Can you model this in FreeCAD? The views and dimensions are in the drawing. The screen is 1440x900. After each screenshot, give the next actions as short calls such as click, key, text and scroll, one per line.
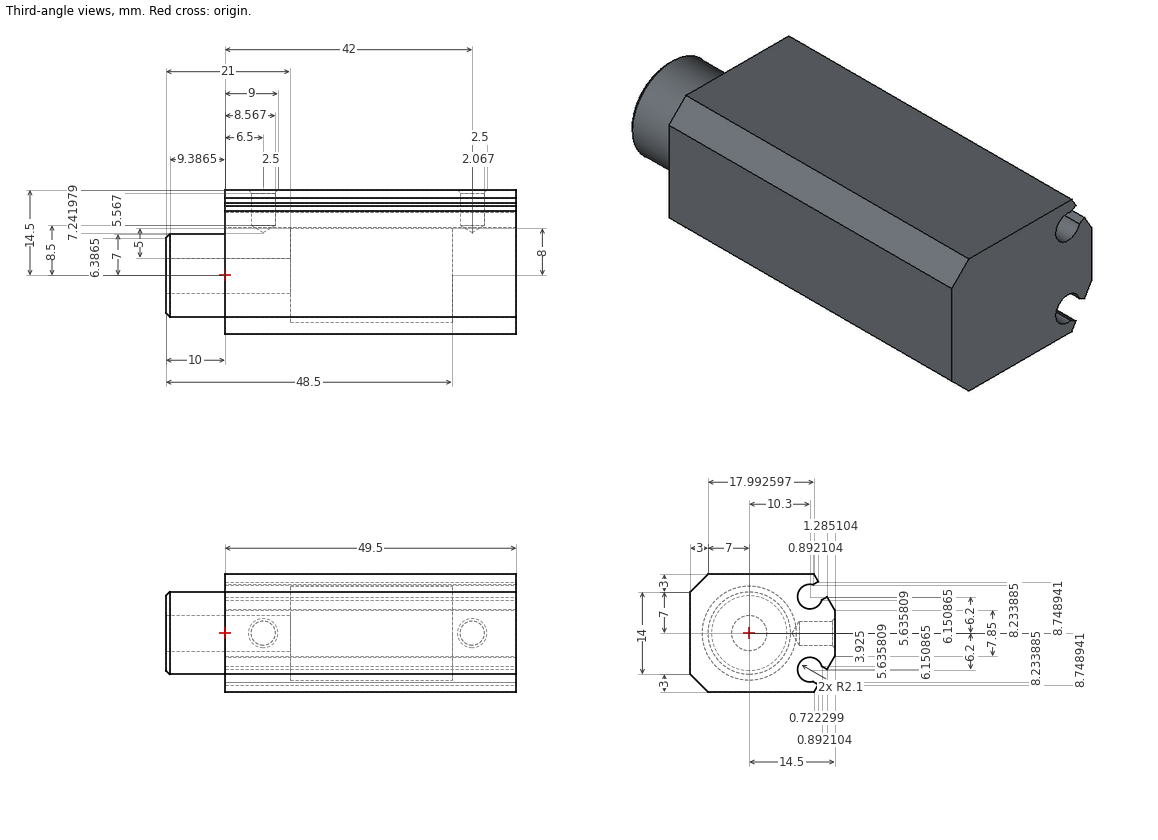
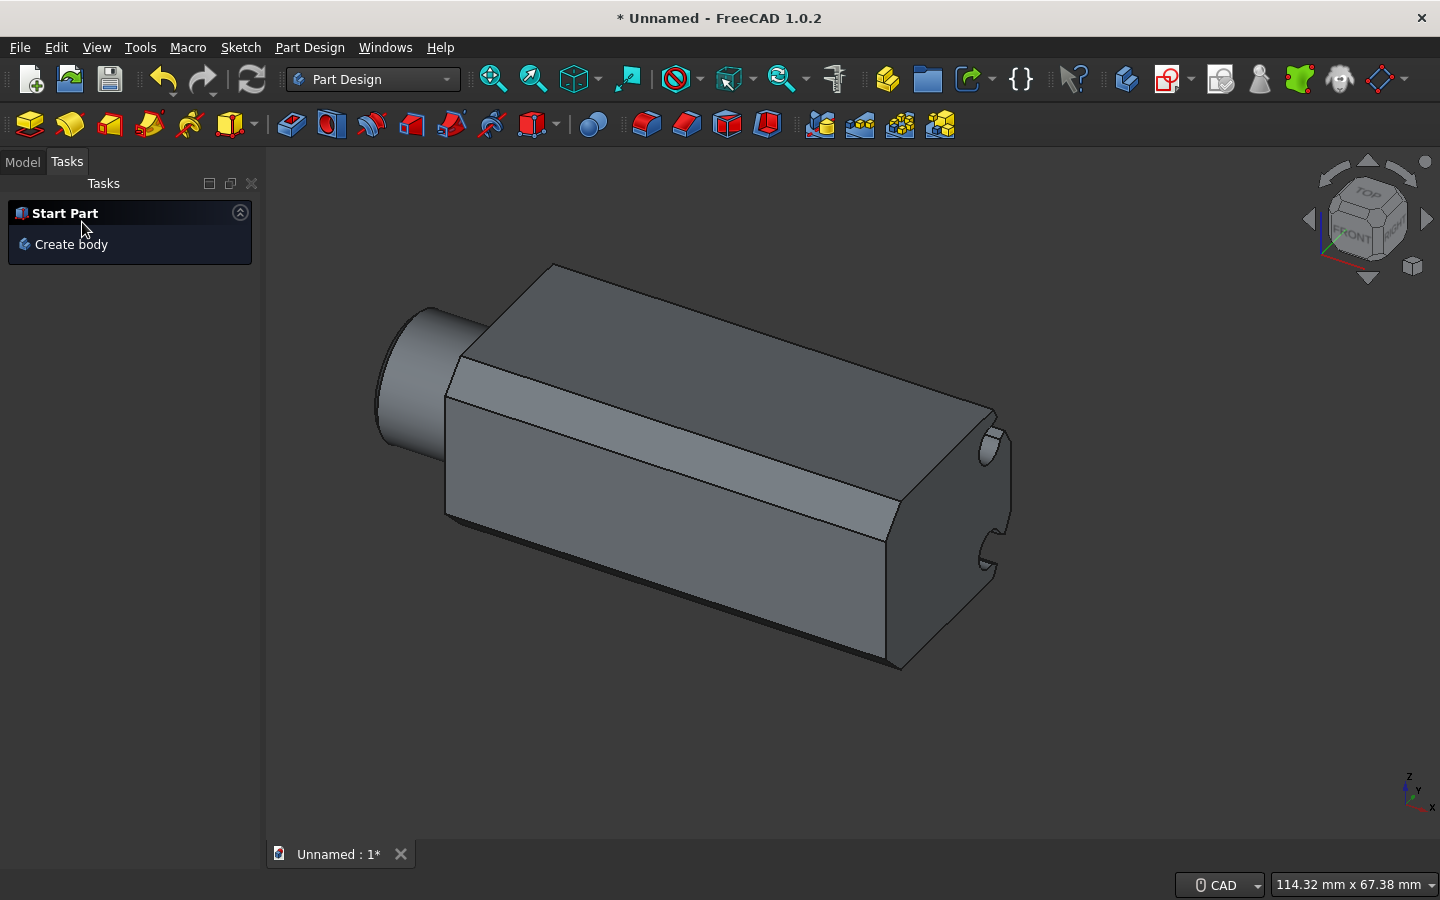
click(1168, 80)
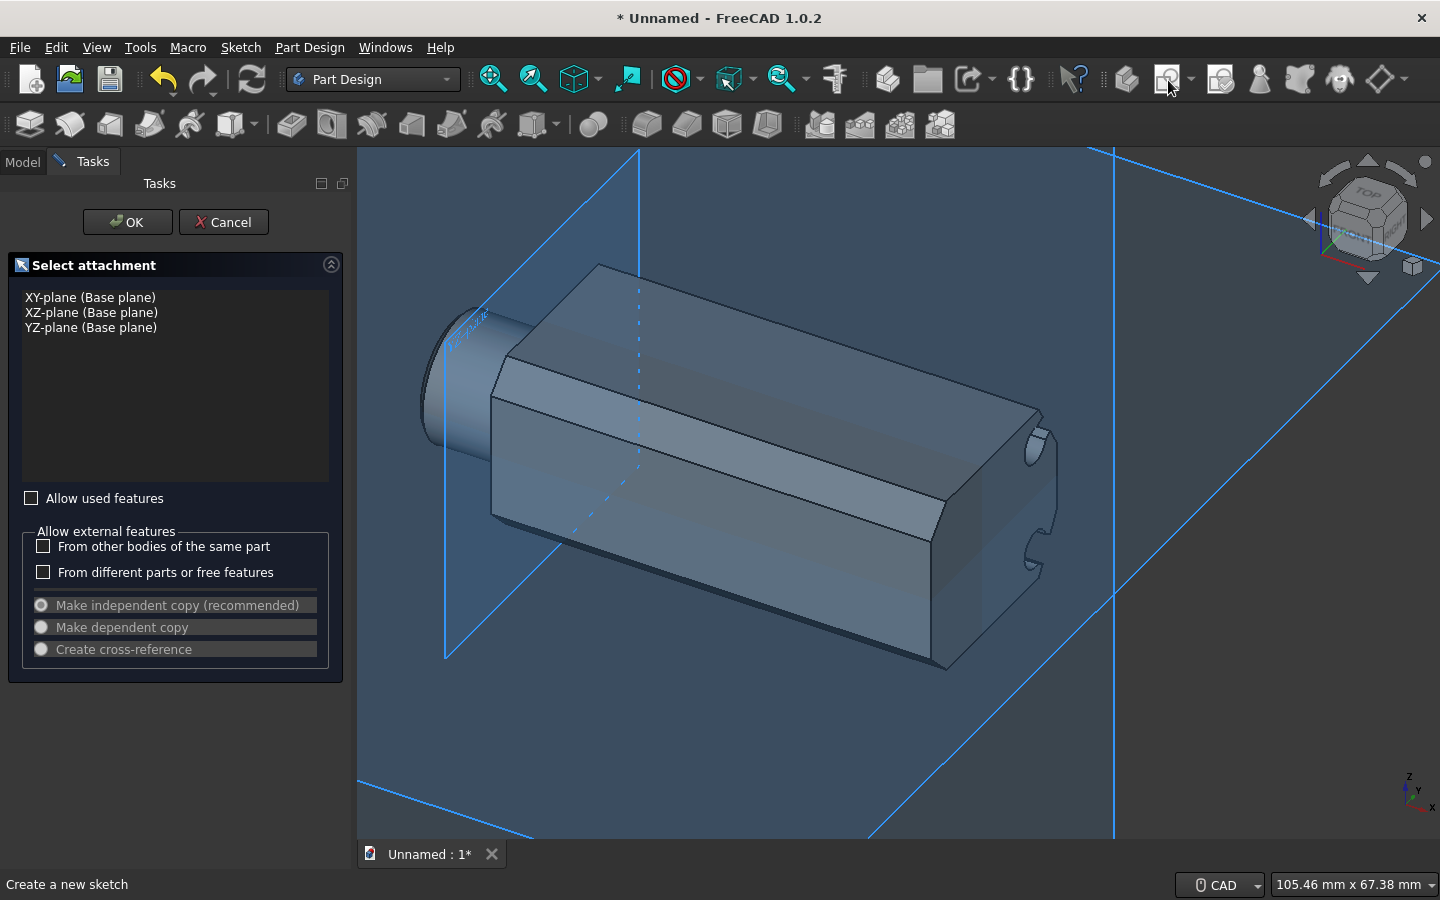
click(82, 298)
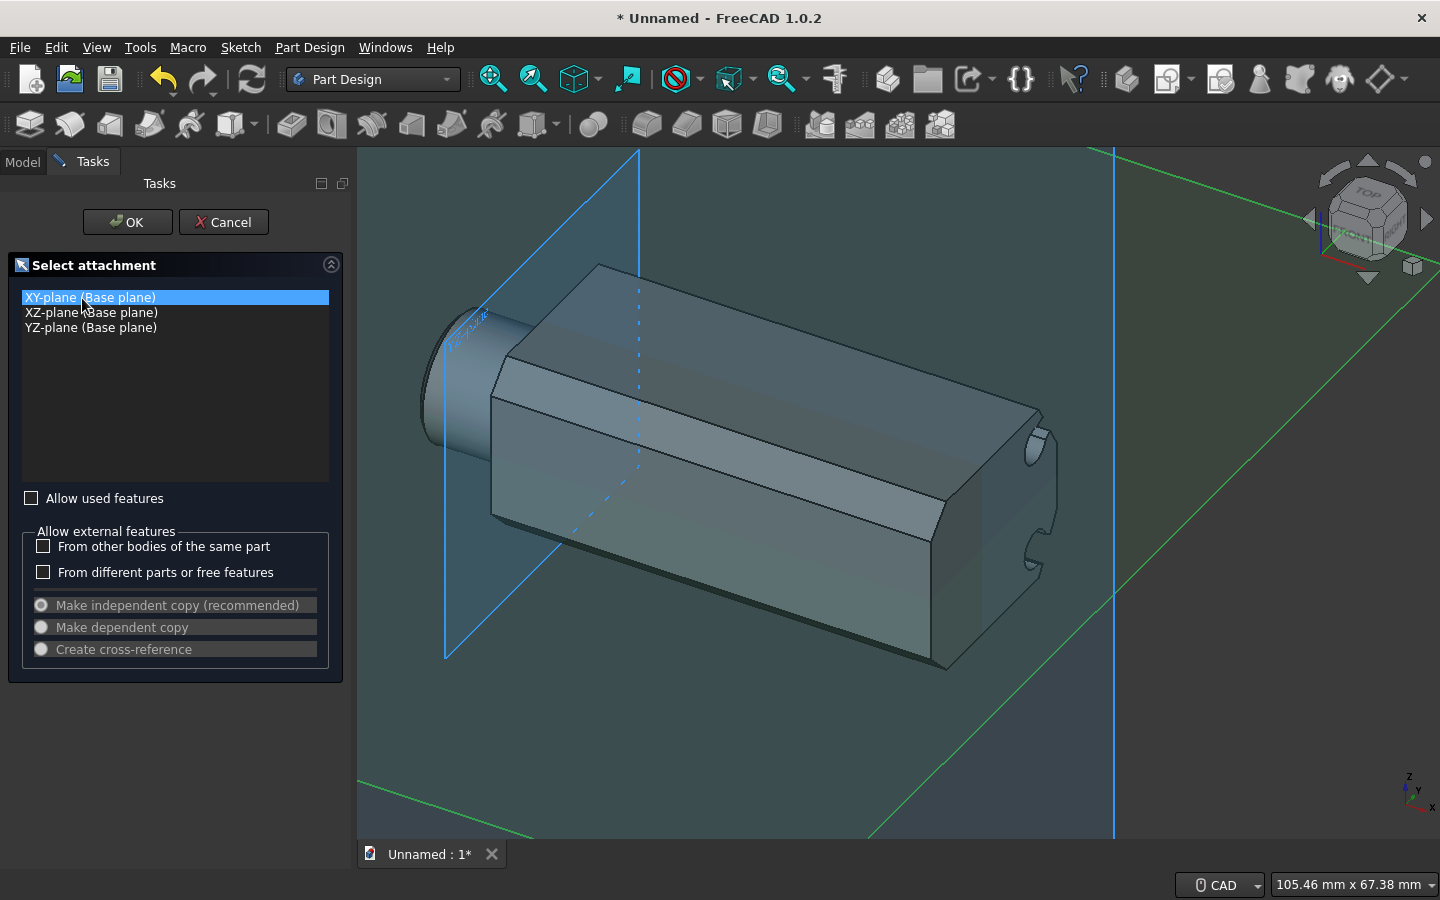
click(128, 222)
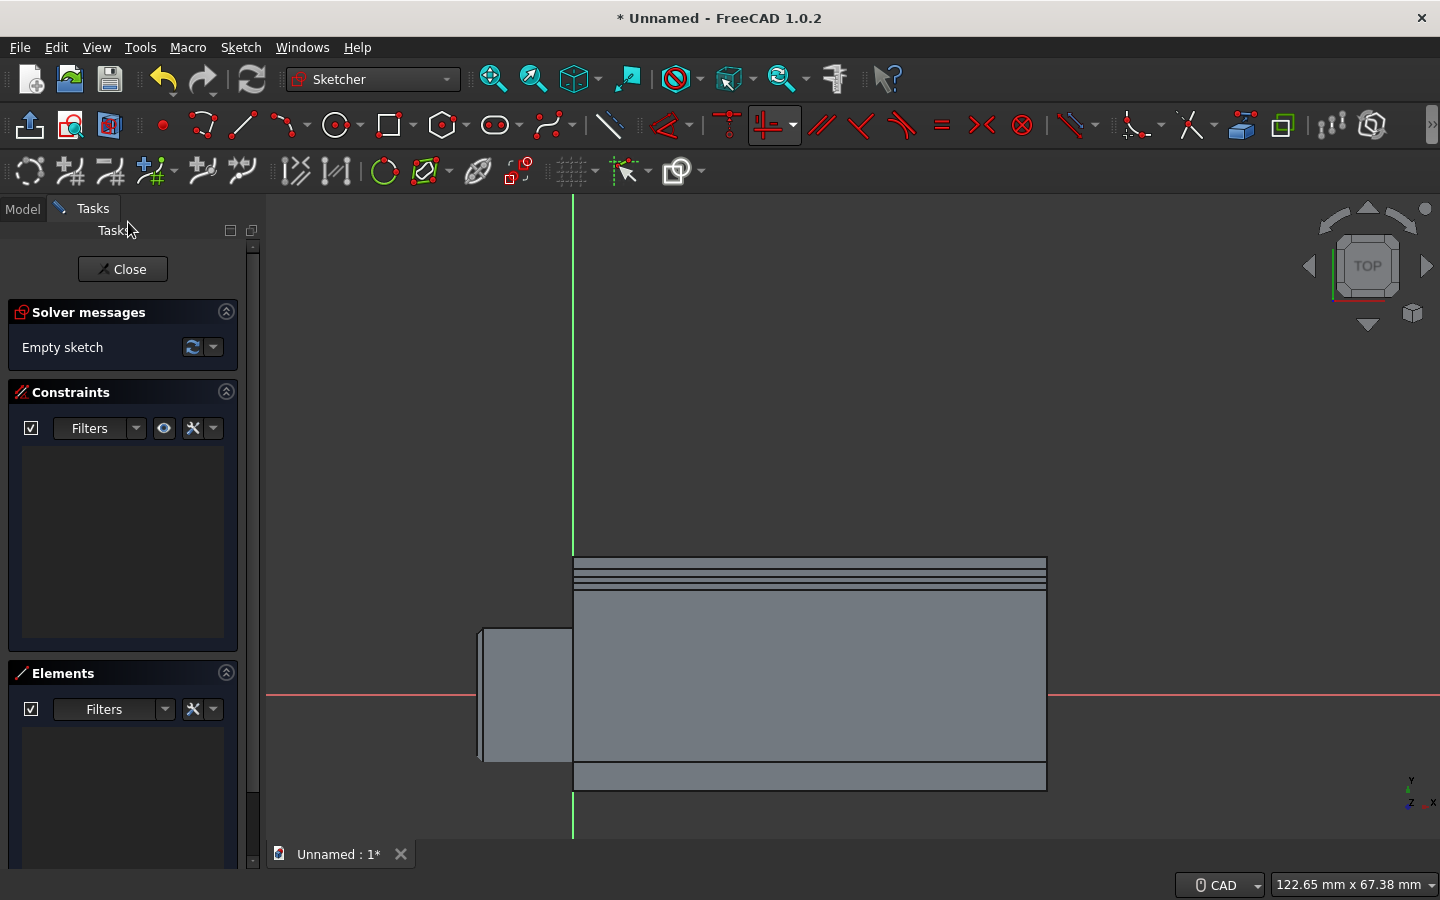
click(110, 126)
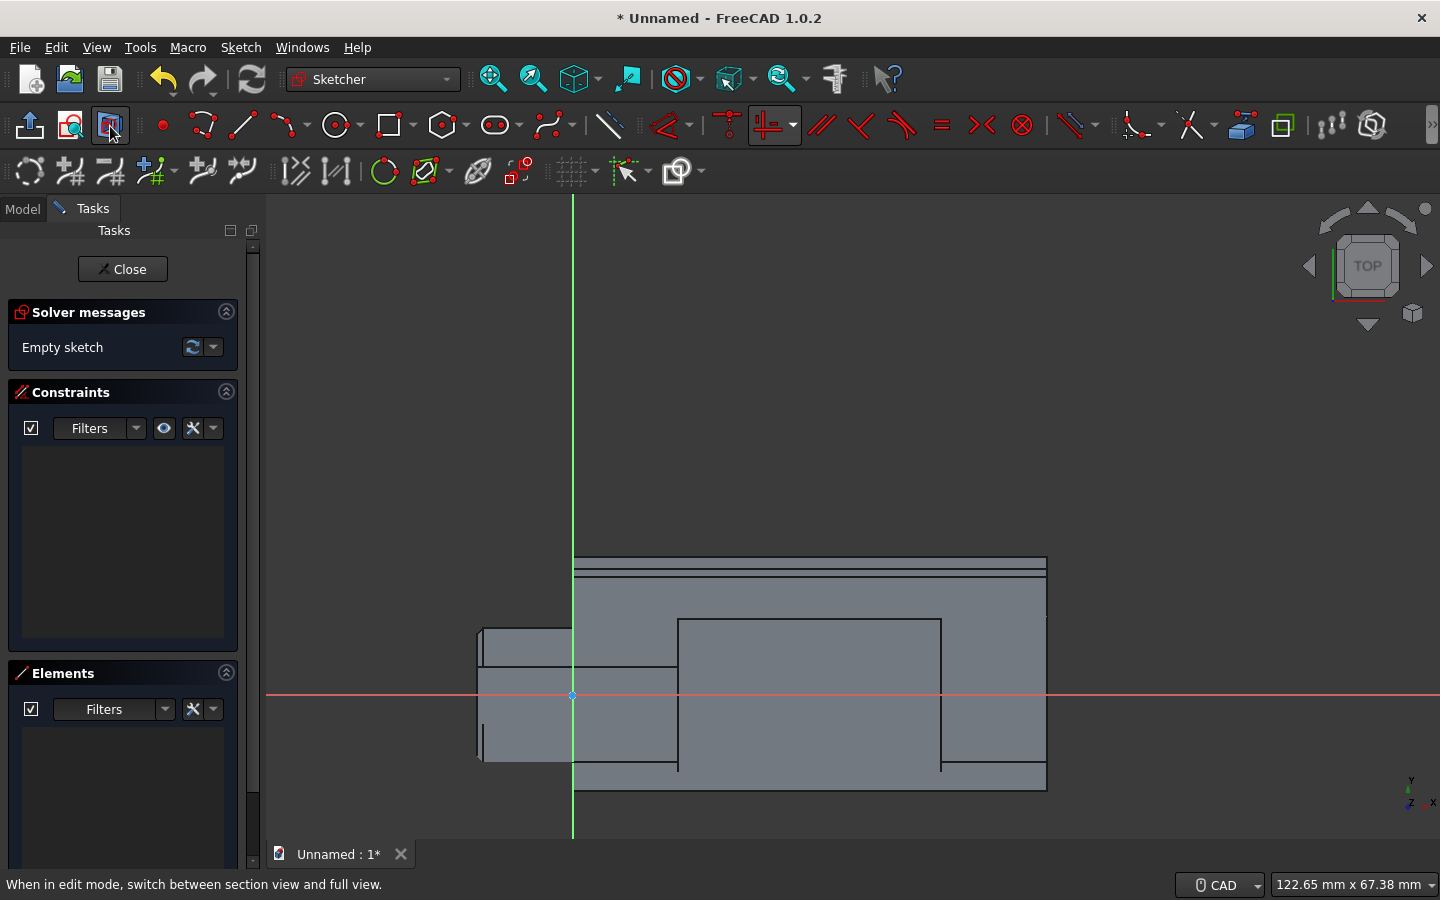
scroll(518, 668, up, 5)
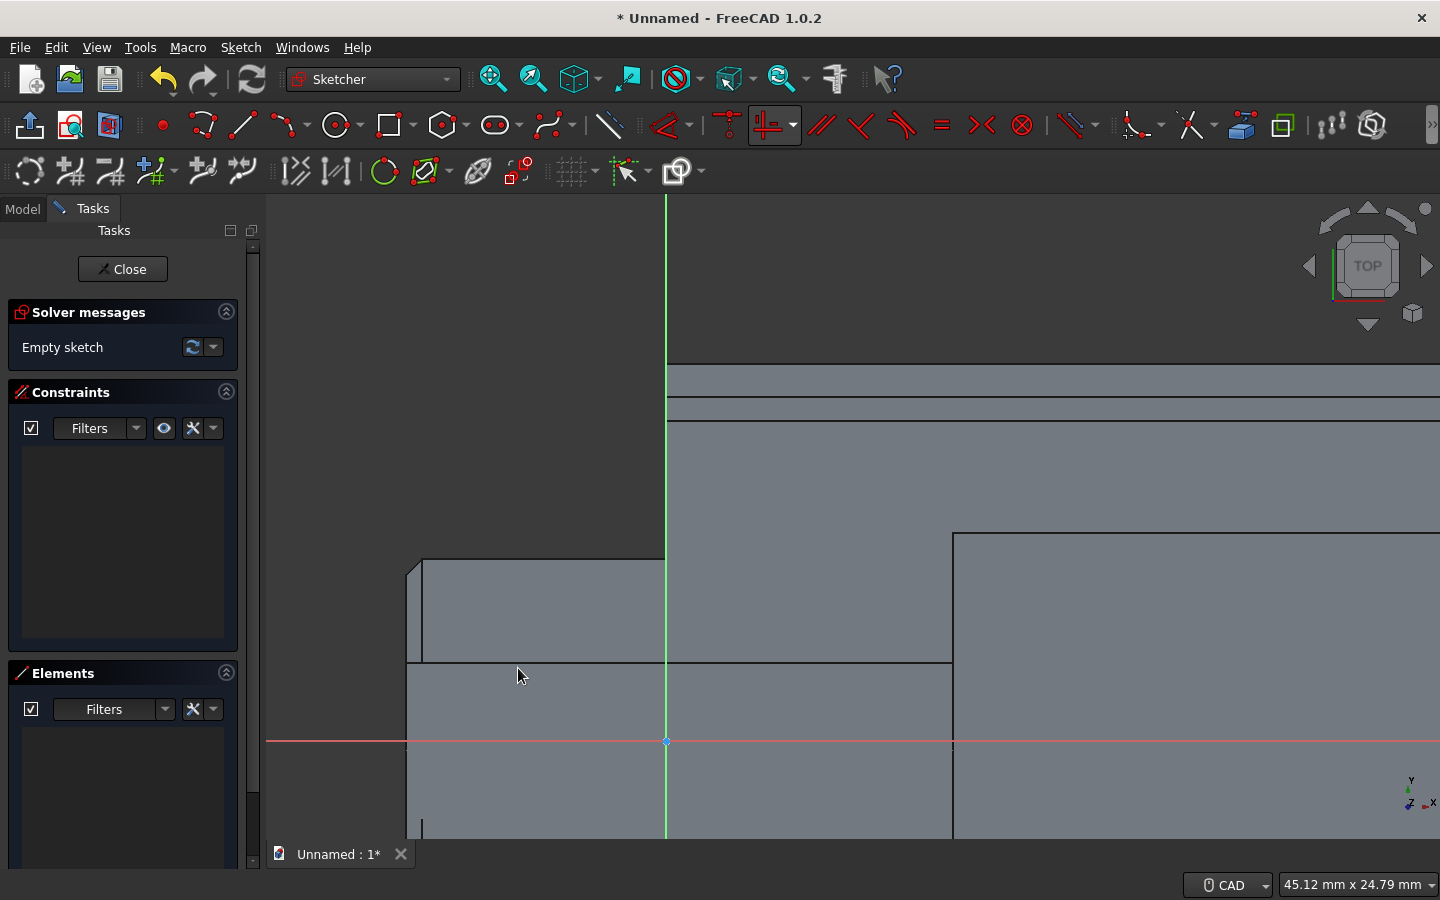
click(204, 126)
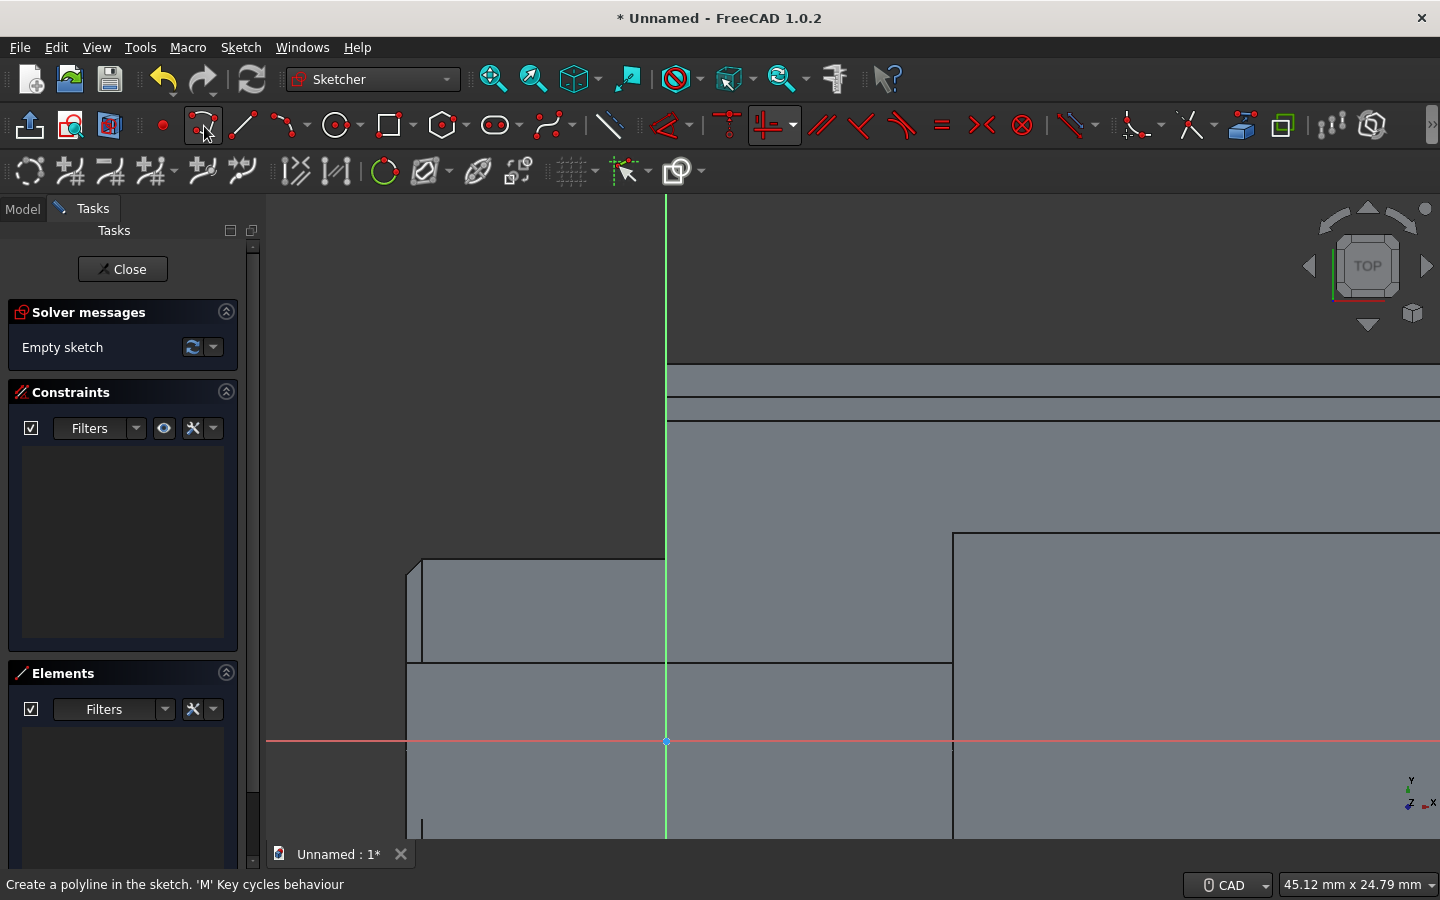
click(836, 552)
click(889, 520)
click(889, 375)
click(901, 364)
click(836, 364)
click(836, 553)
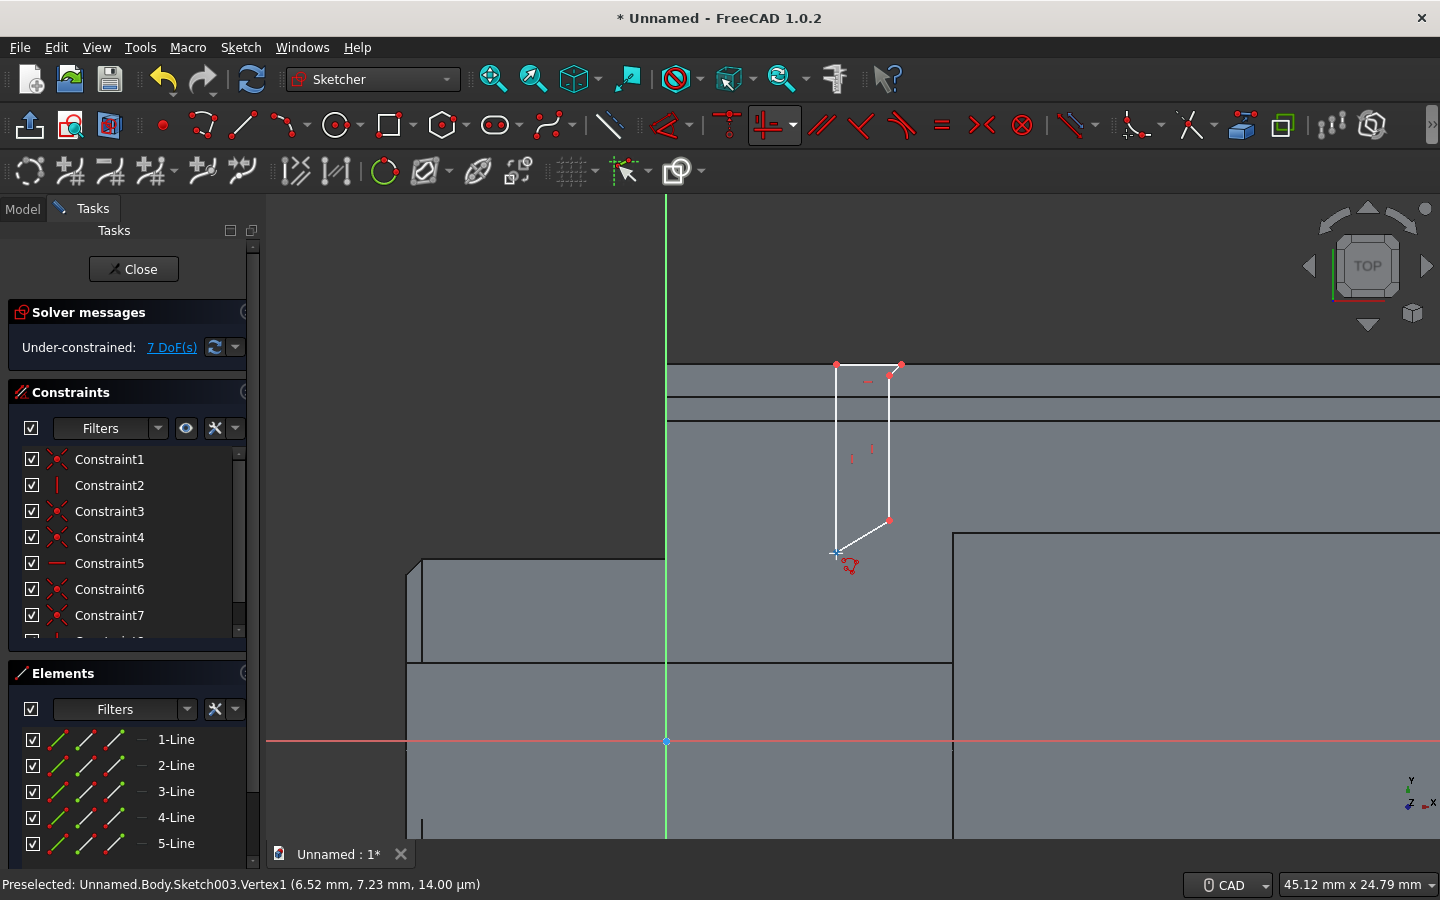
click(244, 126)